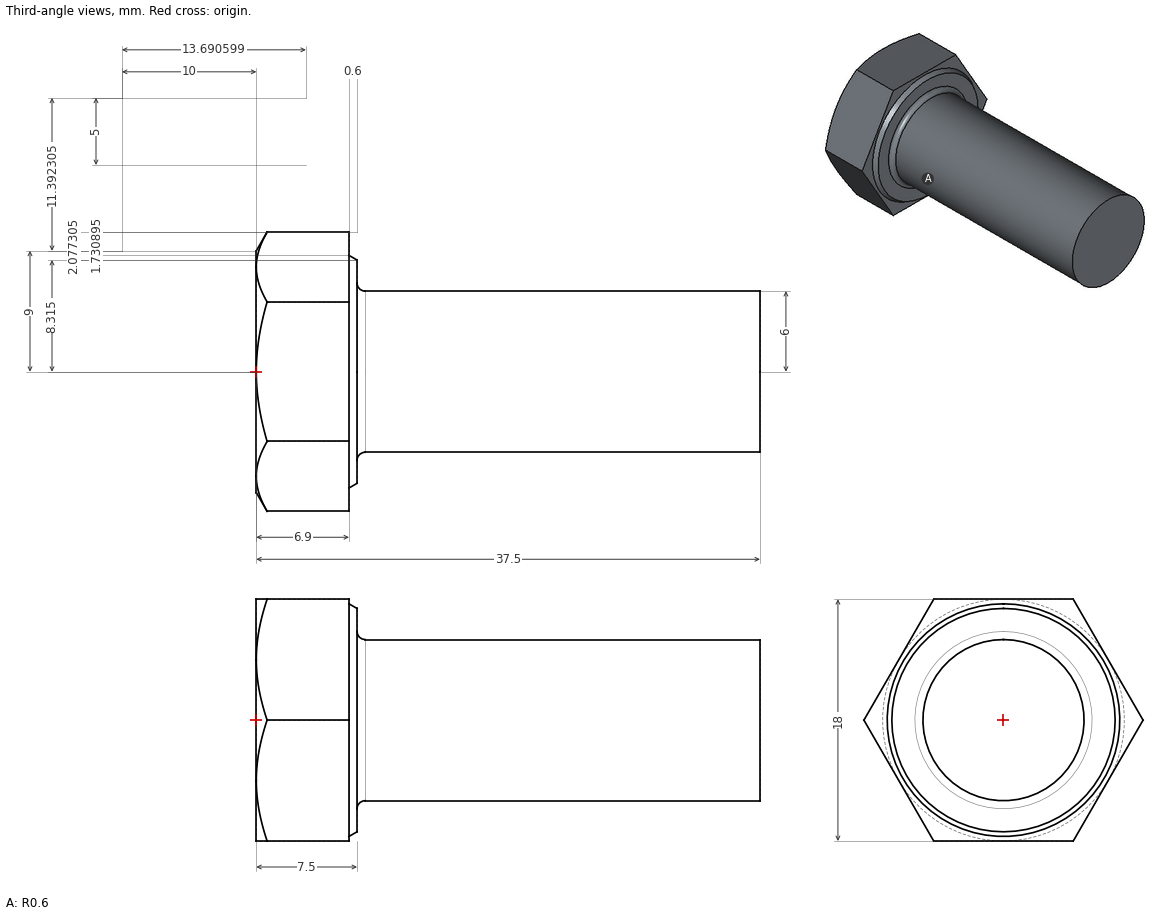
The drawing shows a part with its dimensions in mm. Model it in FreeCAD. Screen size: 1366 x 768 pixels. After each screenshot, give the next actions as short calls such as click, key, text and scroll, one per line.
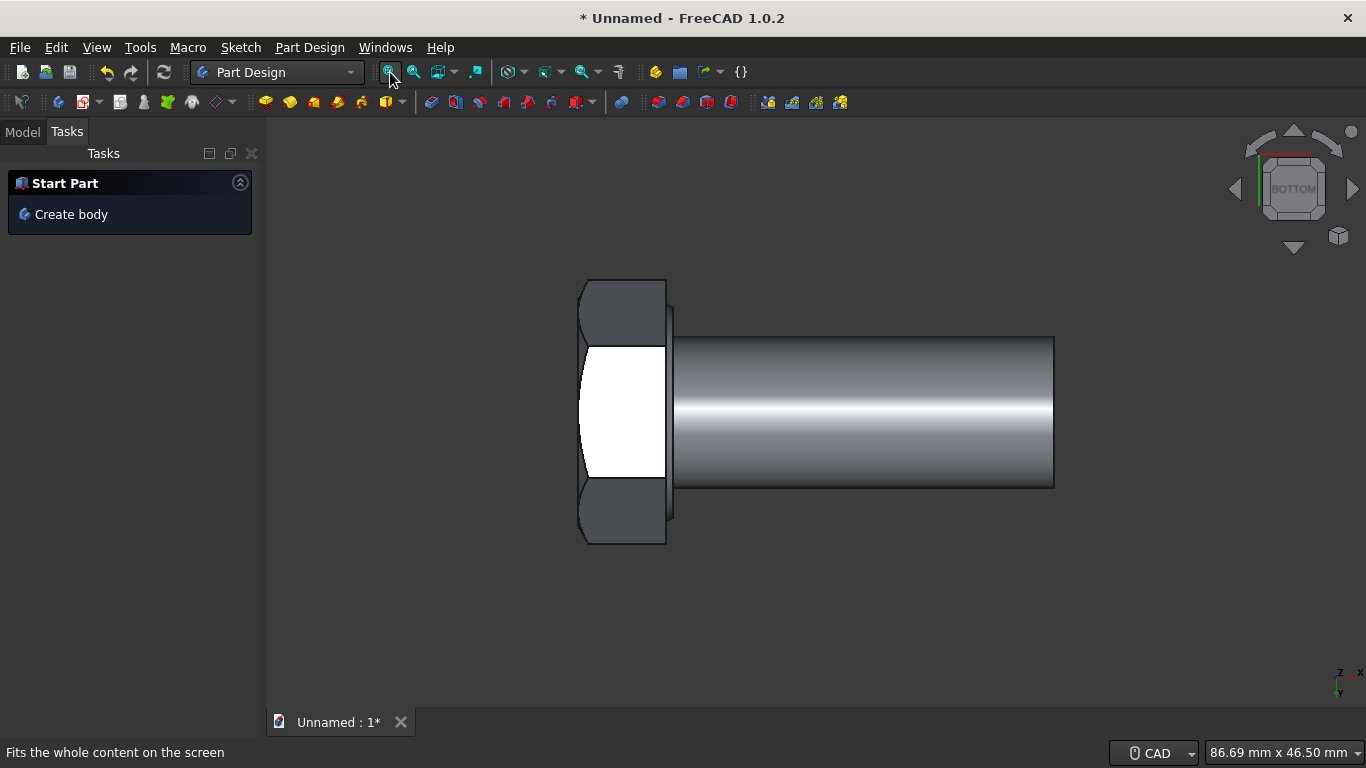
key(v)
key(f)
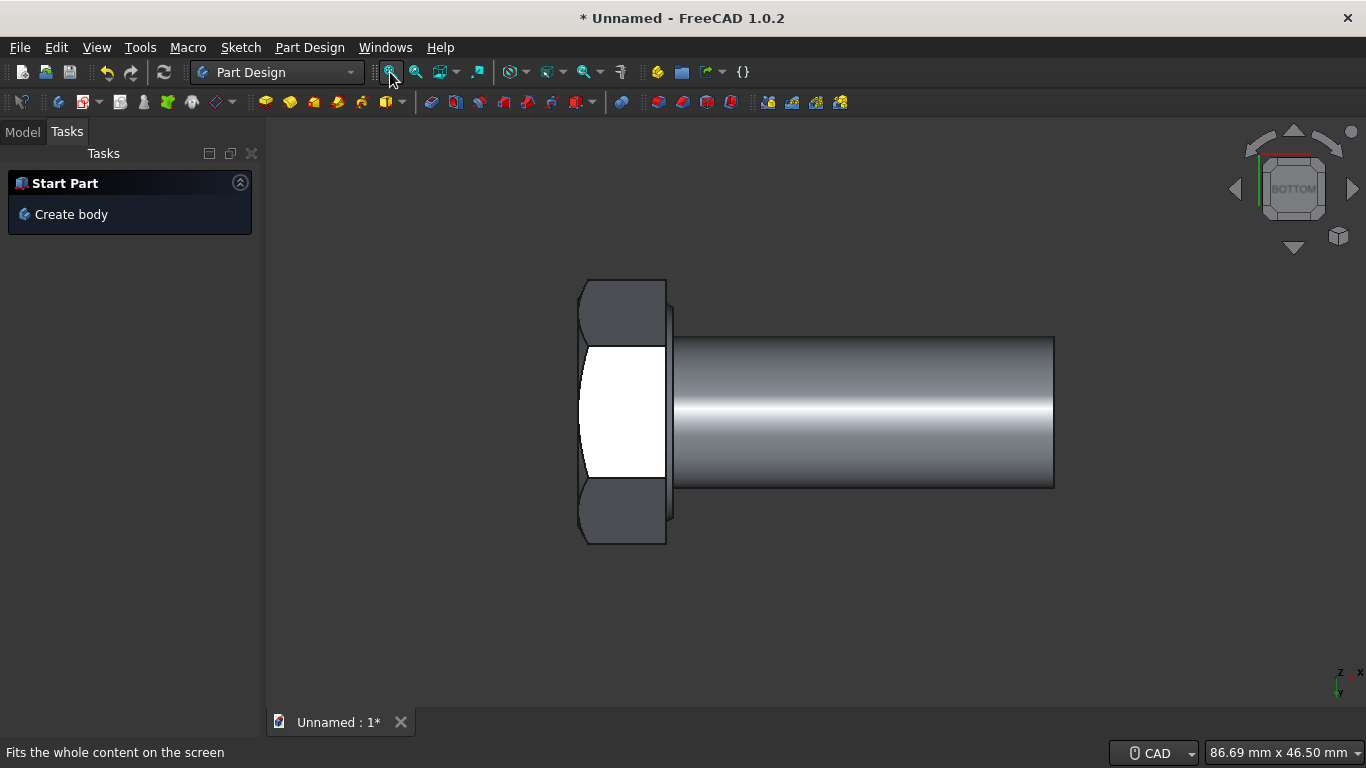
key(4)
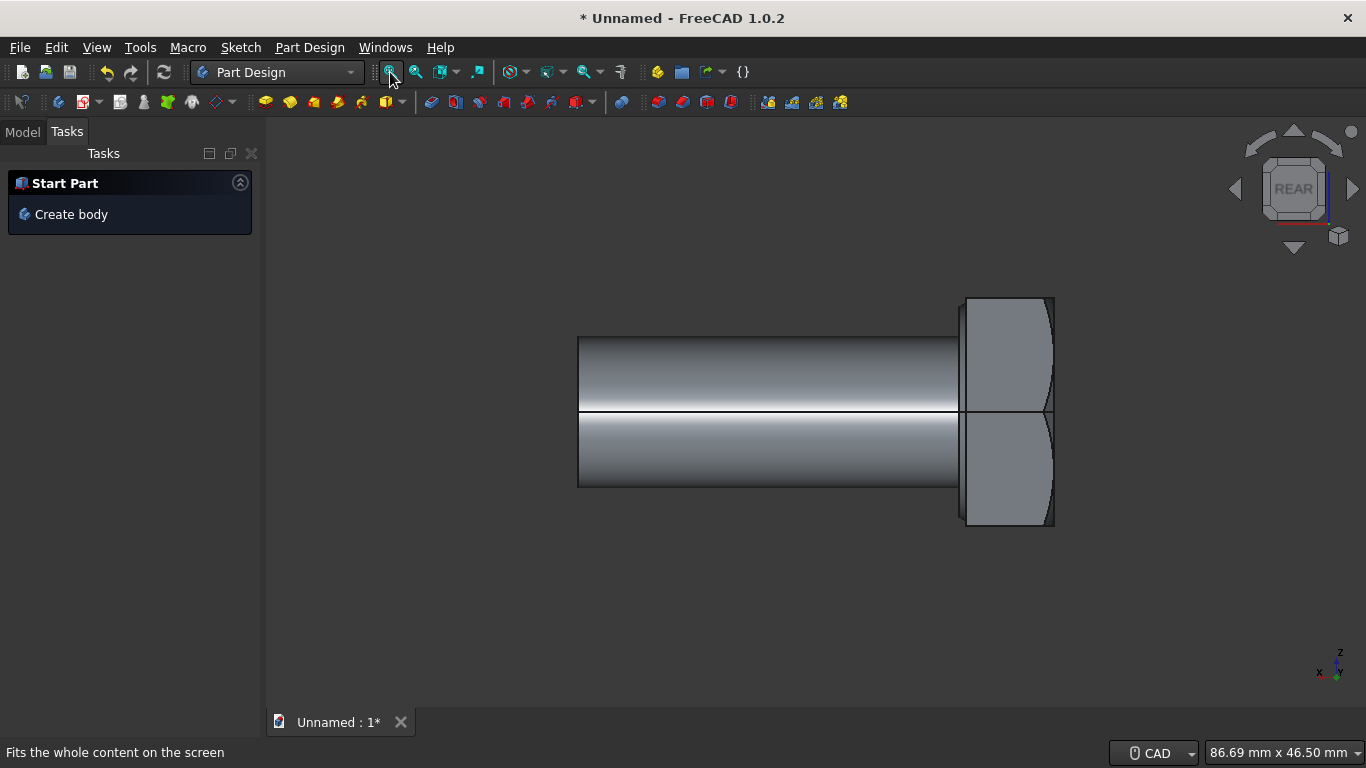
click(392, 72)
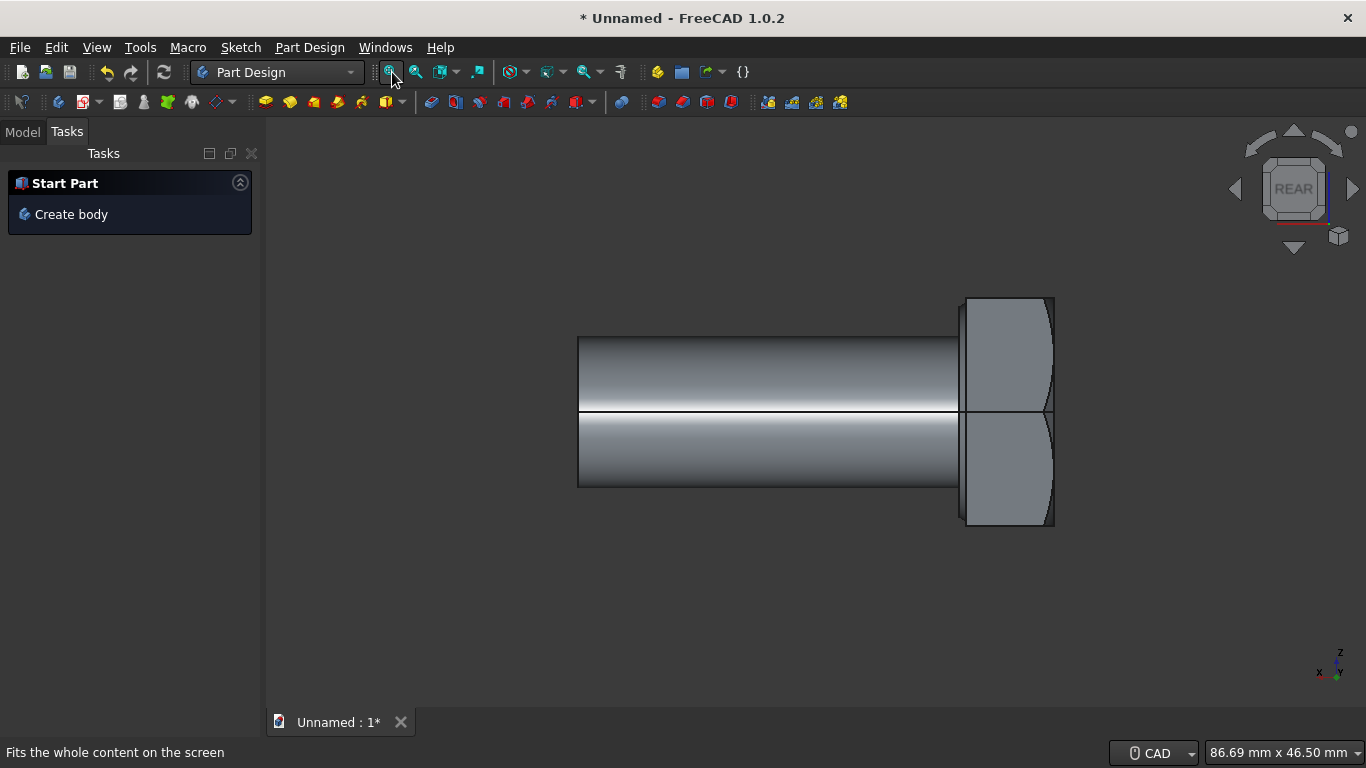
key(6)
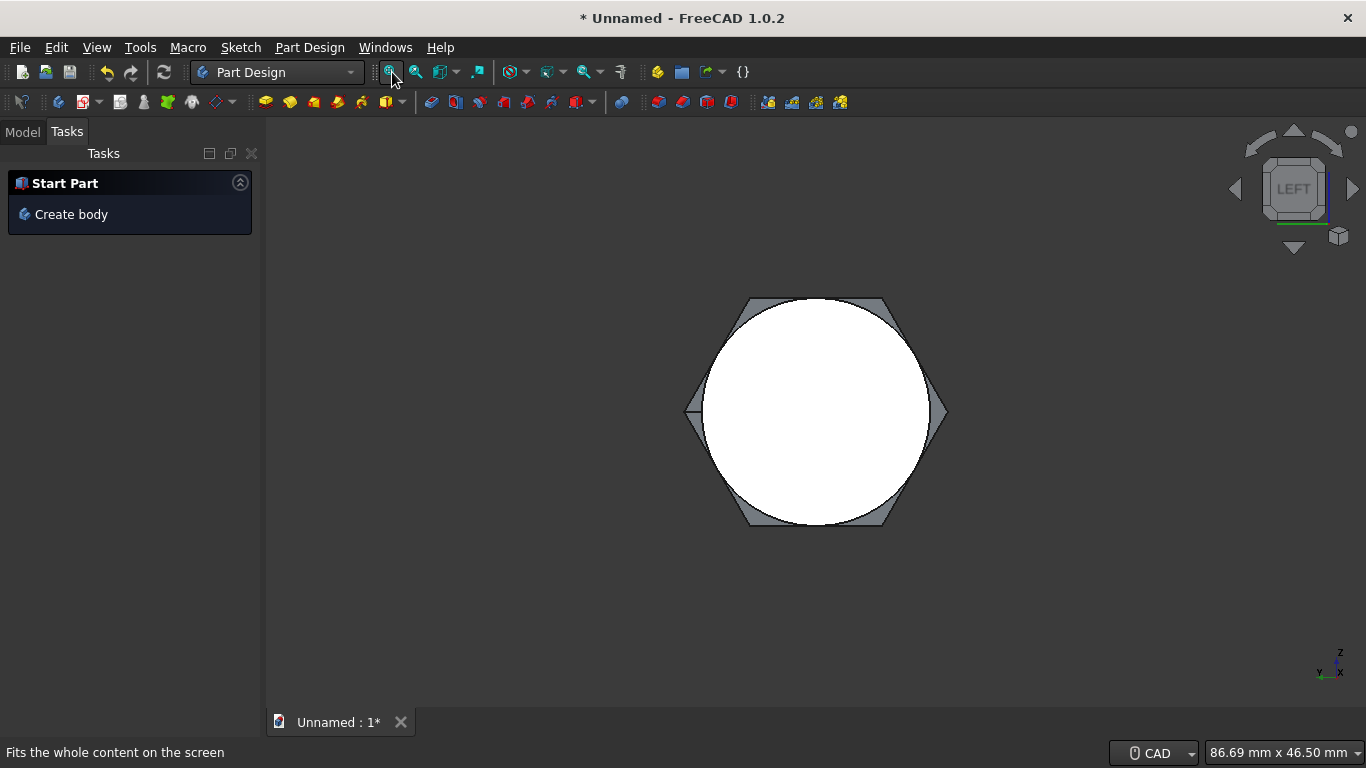
click(392, 72)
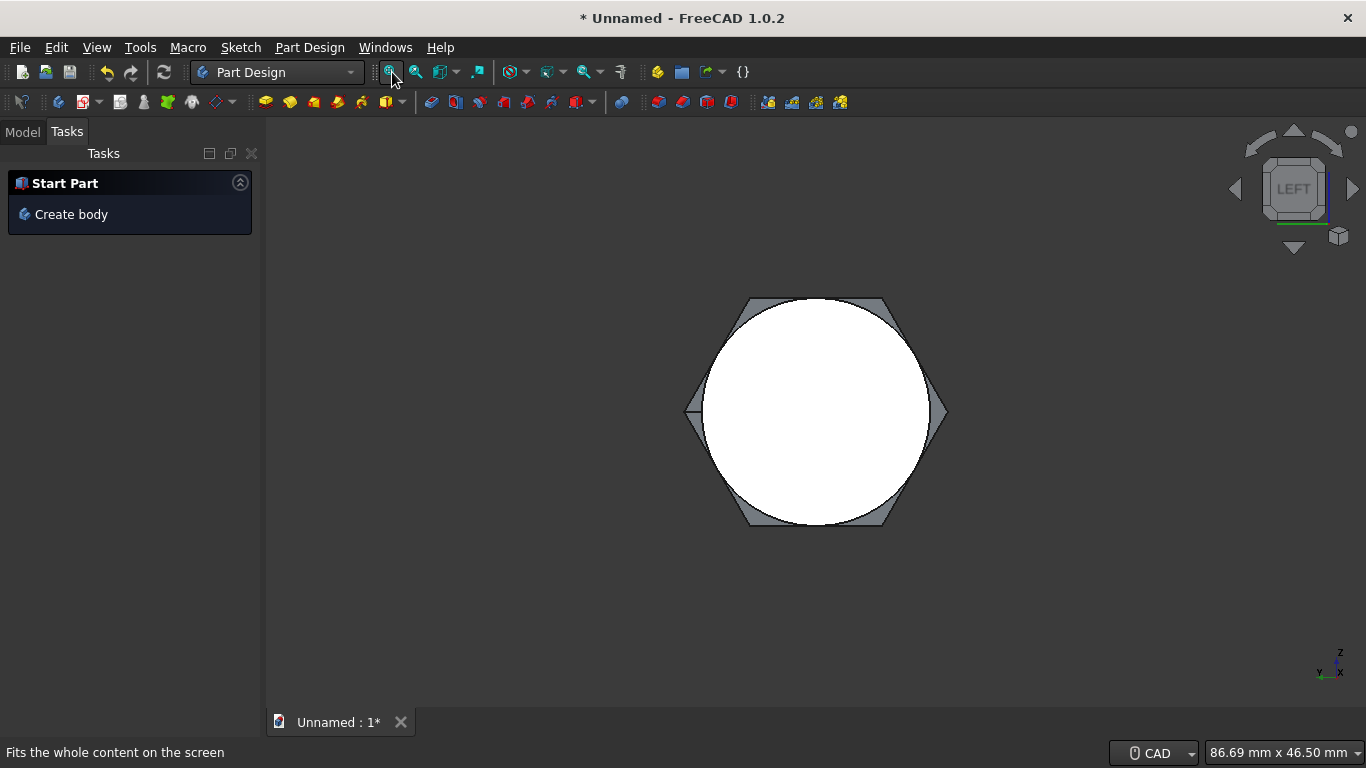
key(v)
key(3)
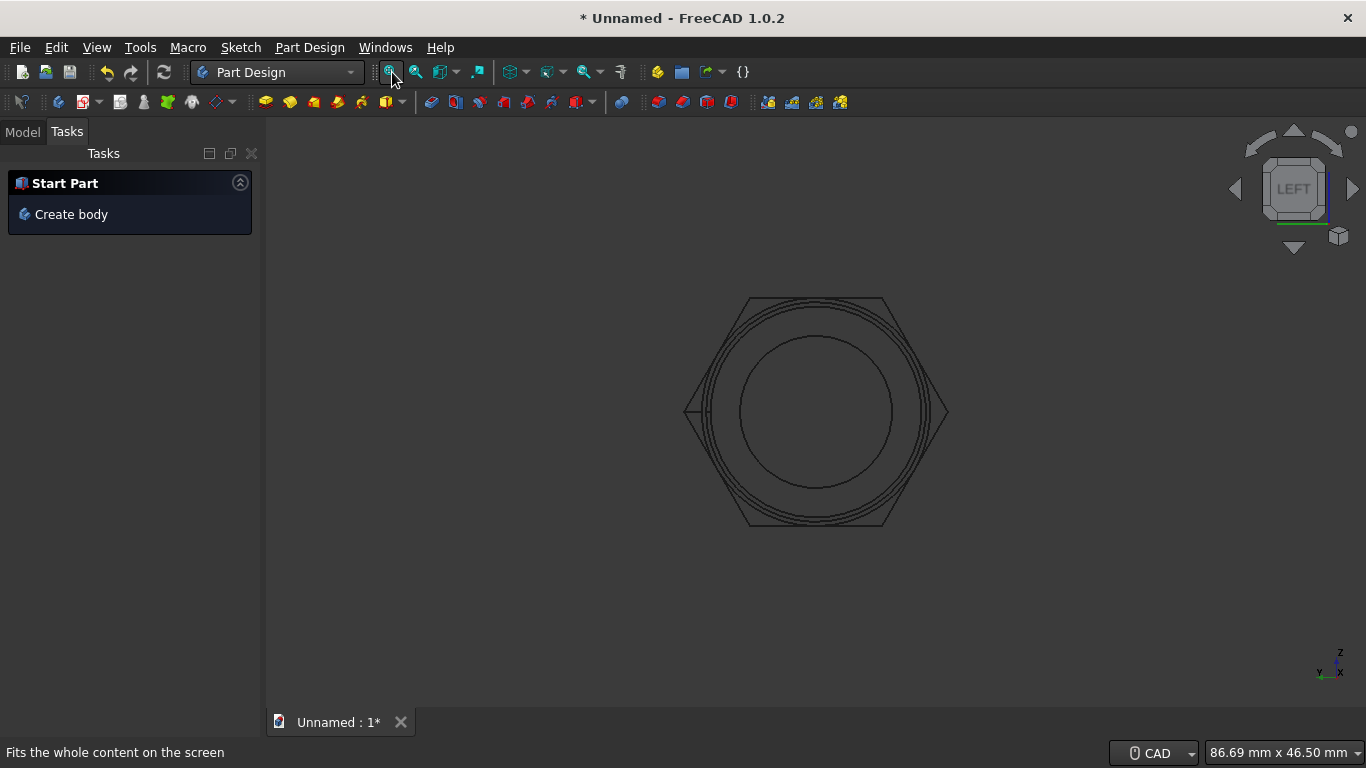
key(0)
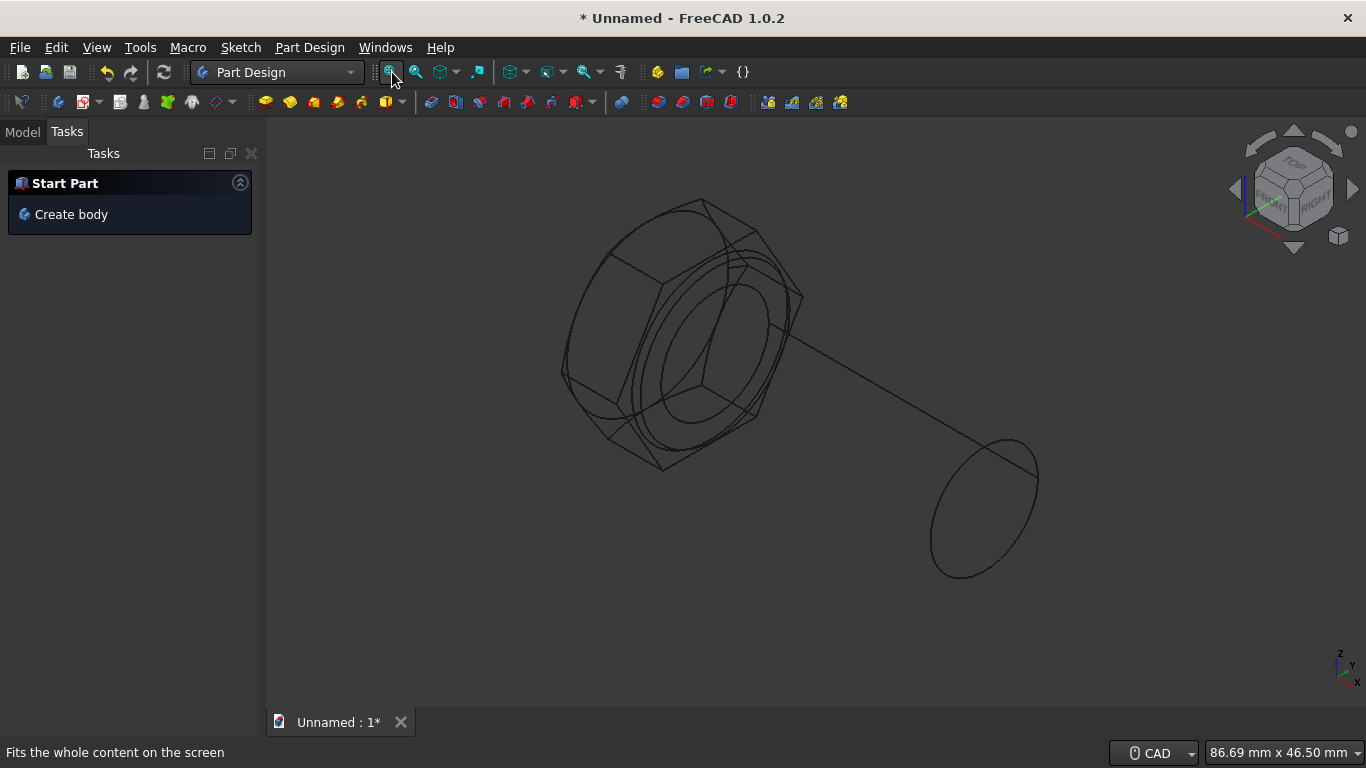
click(661, 384)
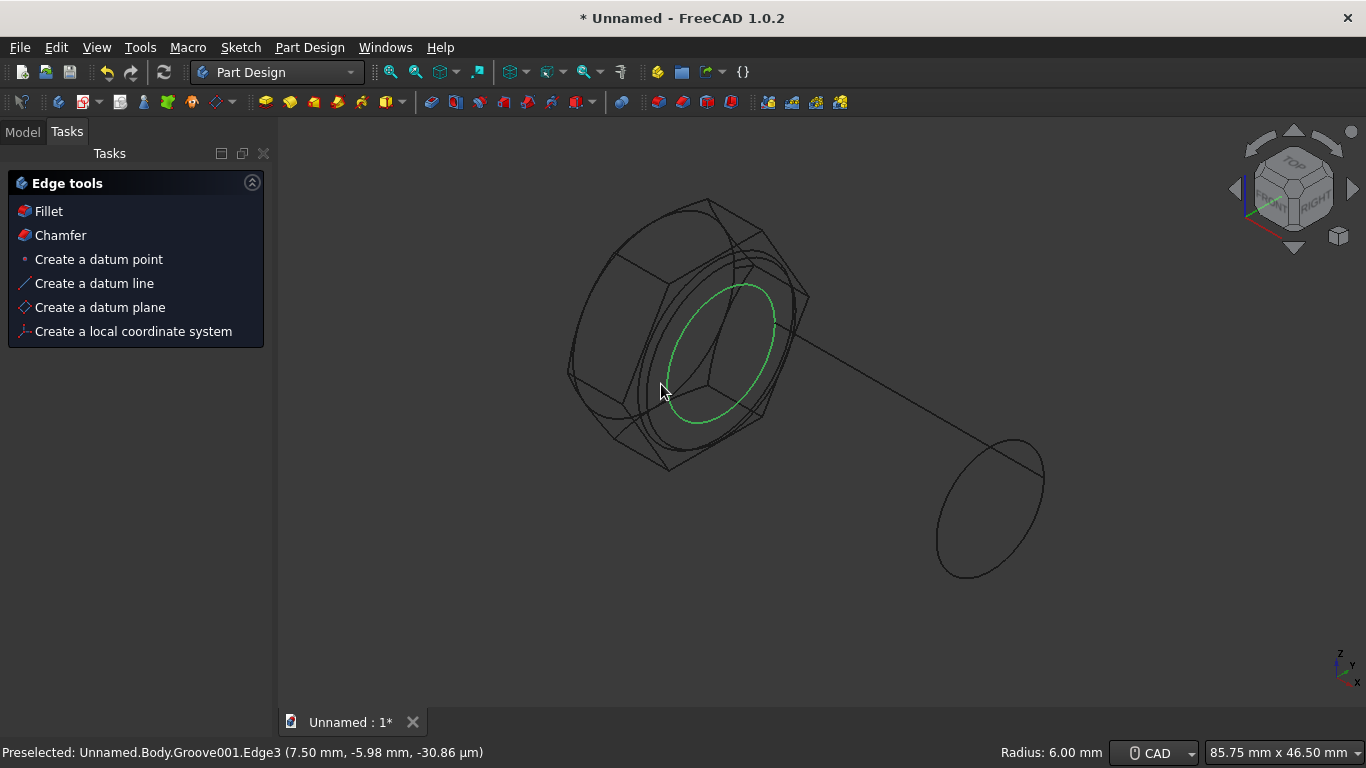
key(v)
key(1)